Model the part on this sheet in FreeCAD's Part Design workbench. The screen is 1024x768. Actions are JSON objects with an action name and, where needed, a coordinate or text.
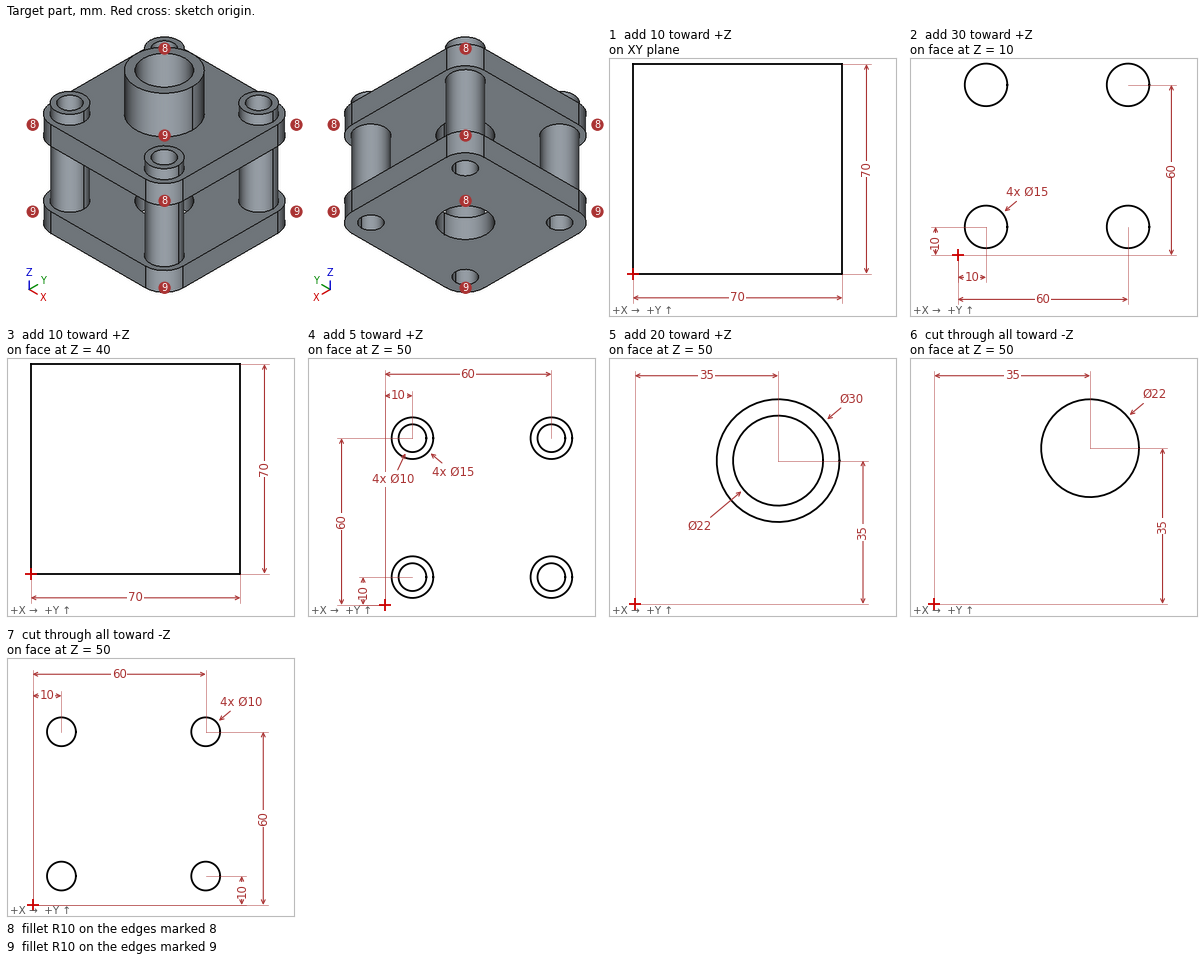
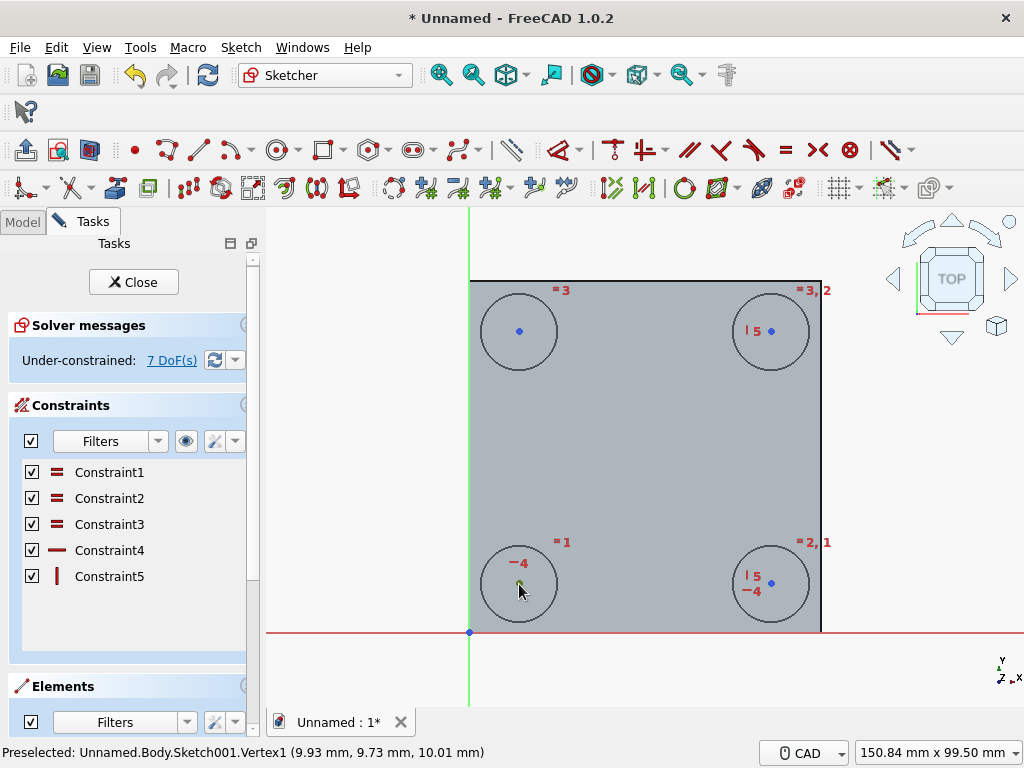
{"action": "left_click", "coordinate": [519, 332]}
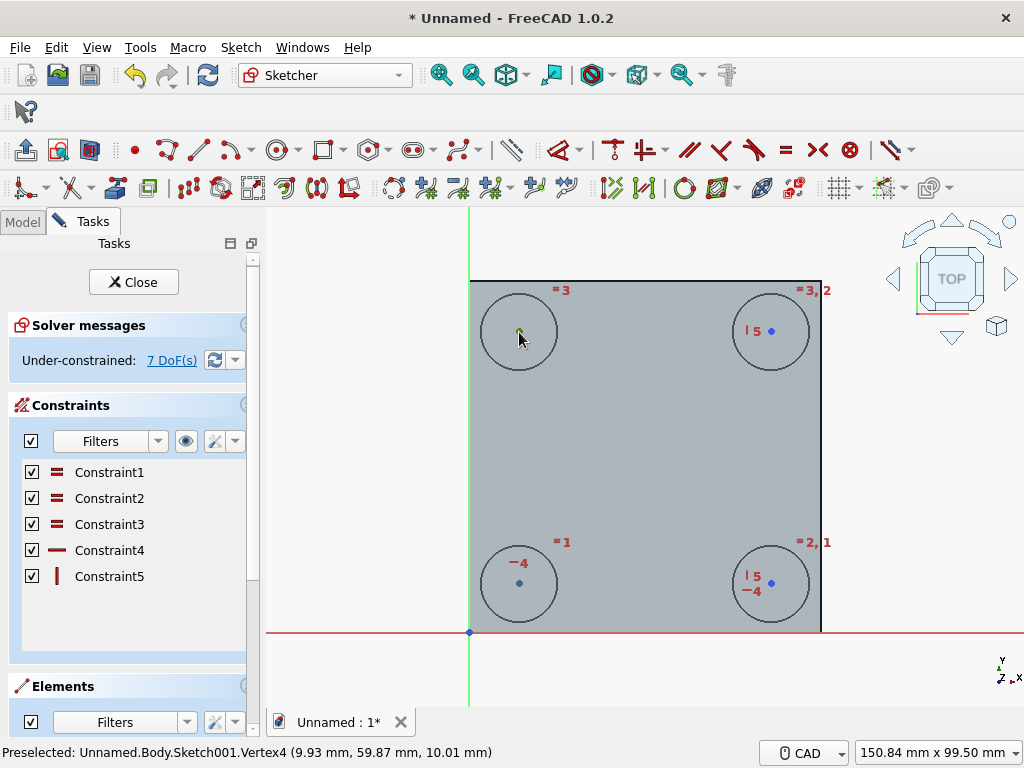
{"action": "key", "text": "v"}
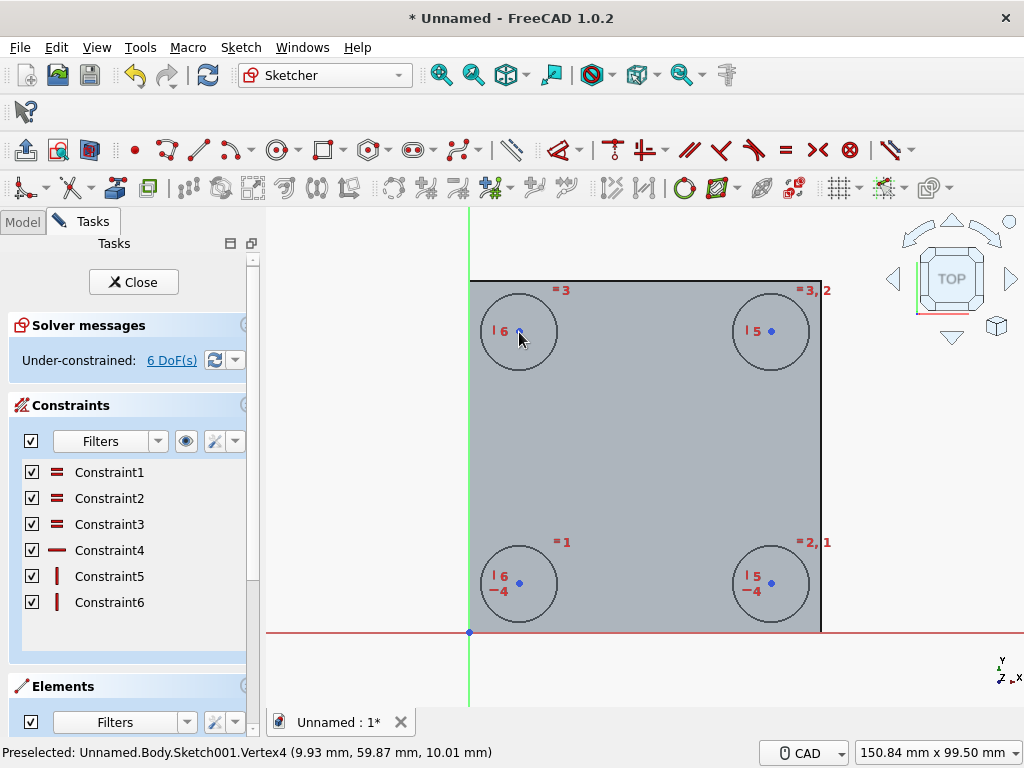
{"action": "left_click", "coordinate": [771, 332]}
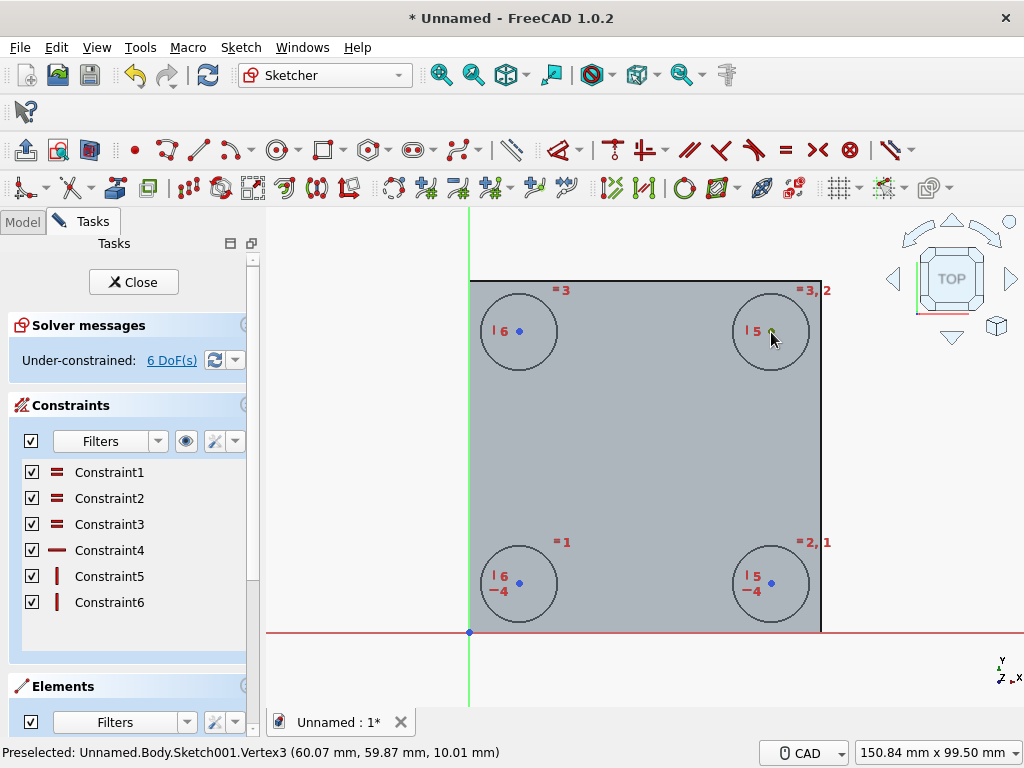
{"action": "left_click", "coordinate": [519, 332]}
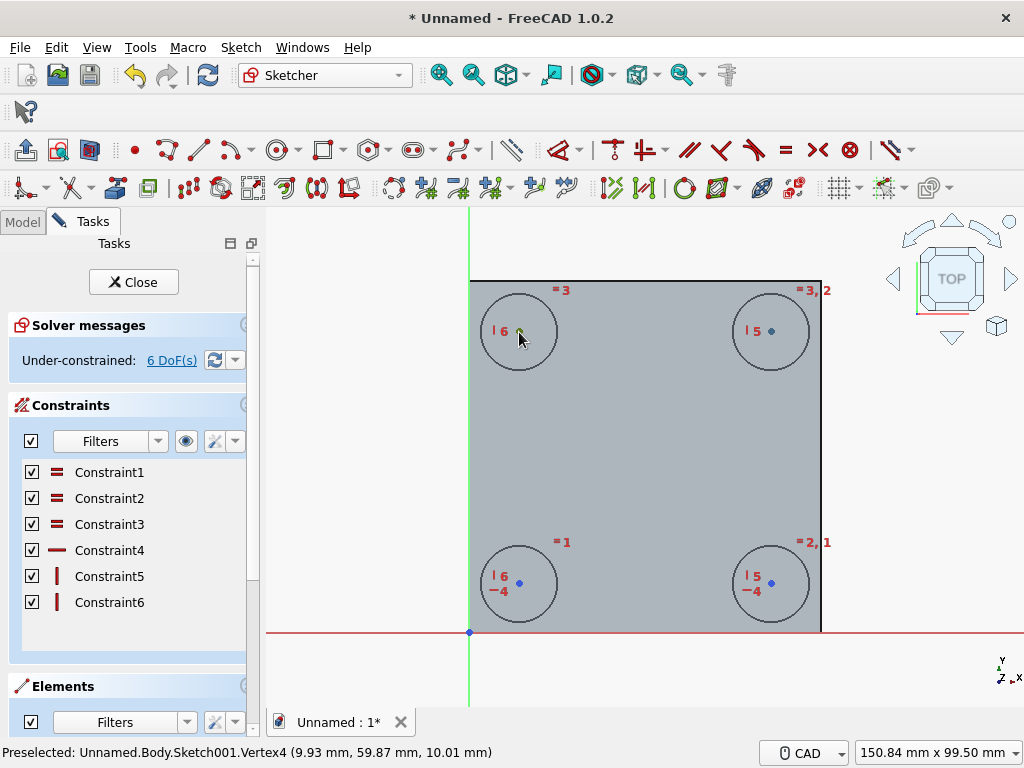
{"action": "key", "text": "h"}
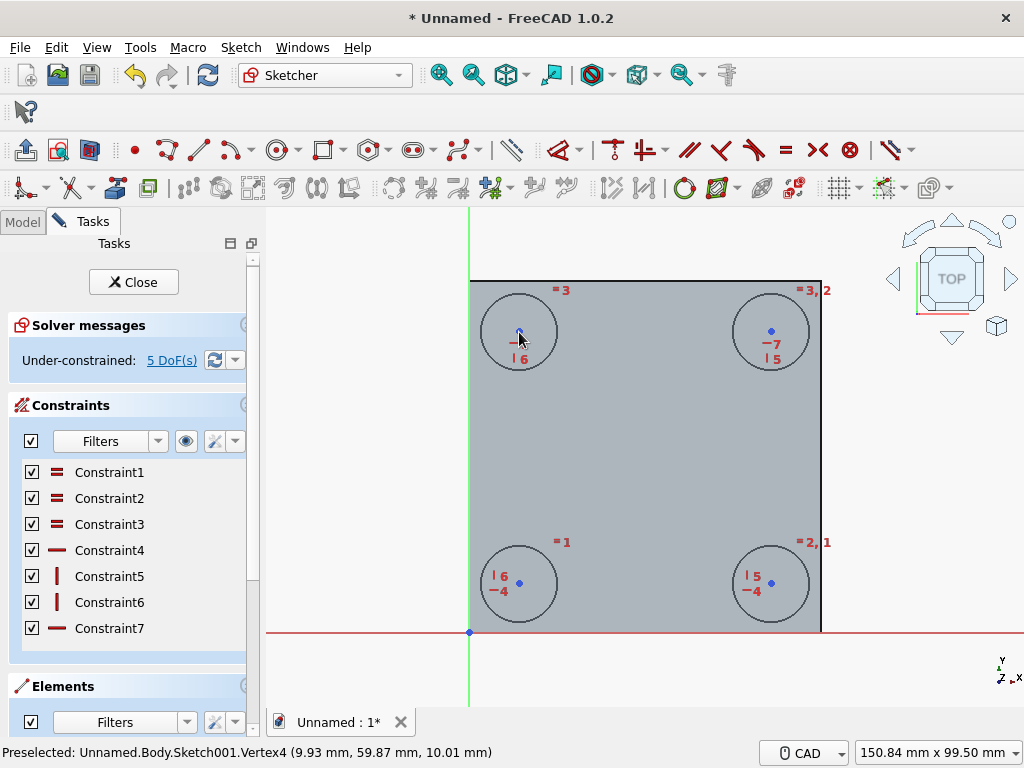
{"action": "key", "text": "d"}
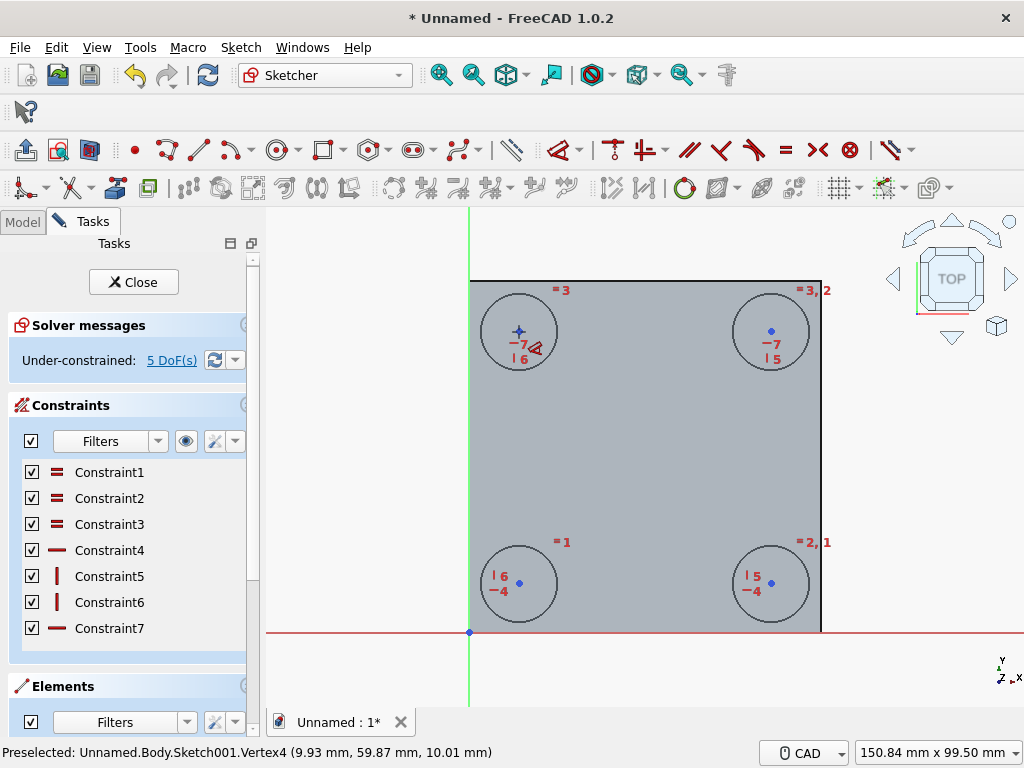
{"action": "left_click", "coordinate": [546, 557]}
{"action": "left_click", "coordinate": [569, 534]}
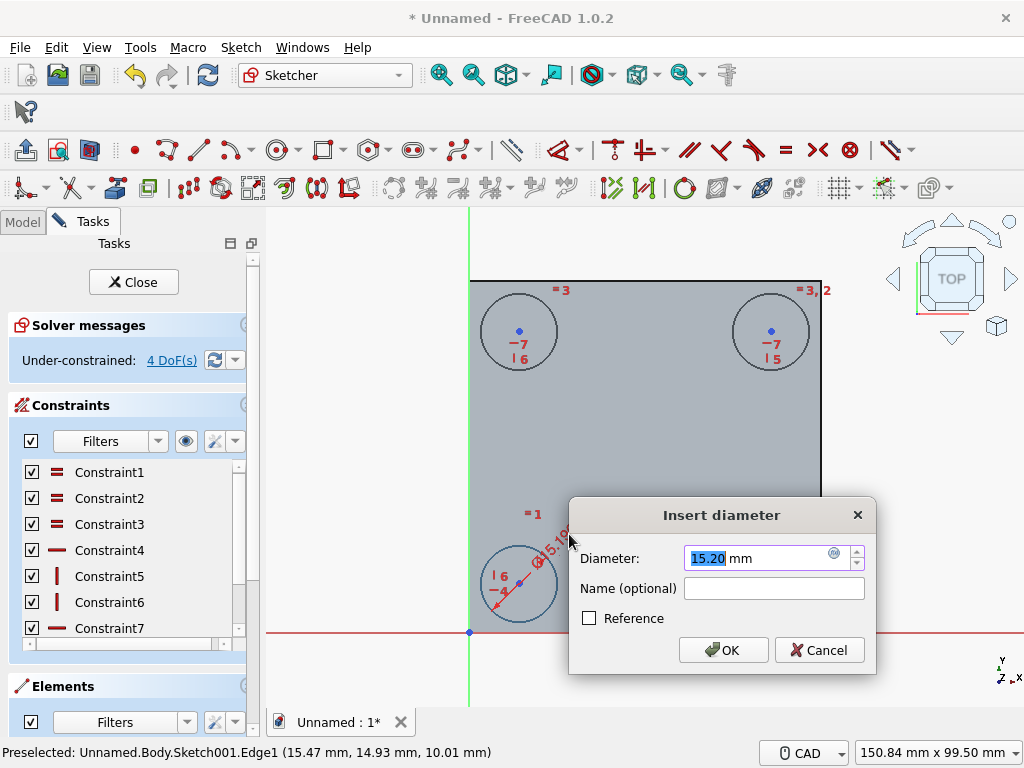
{"action": "type", "text": "15"}
{"action": "key", "text": "Return"}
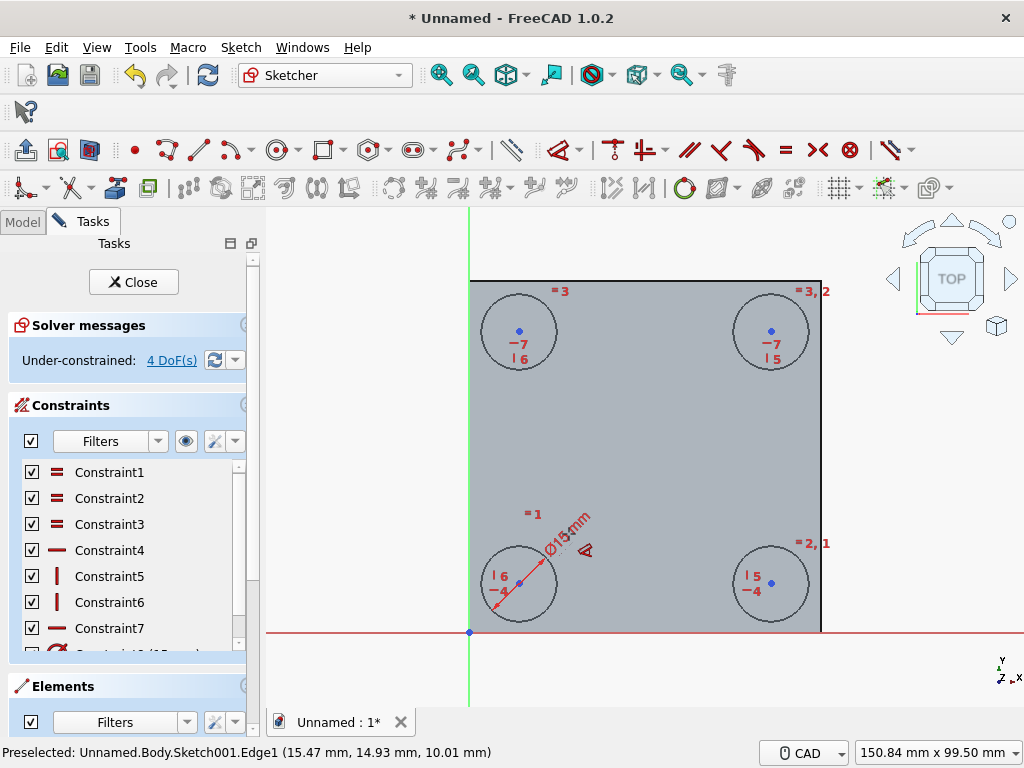
{"action": "left_click", "coordinate": [519, 584]}
{"action": "left_click", "coordinate": [494, 667]}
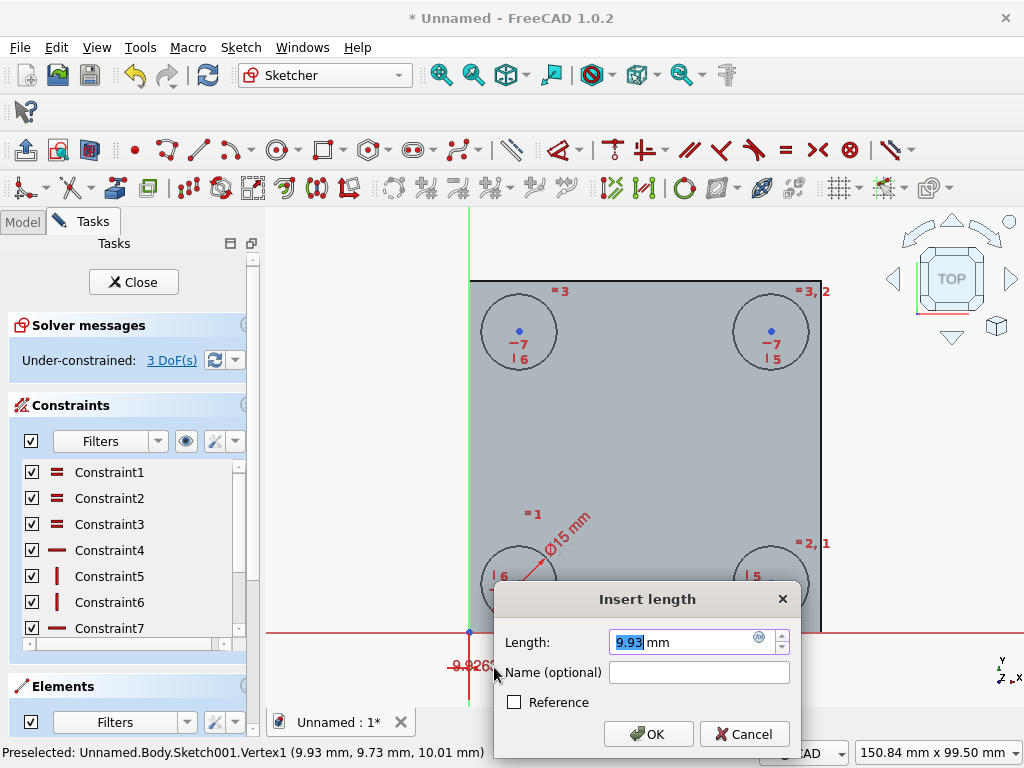
{"action": "type", "text": "10"}
{"action": "key", "text": "Return"}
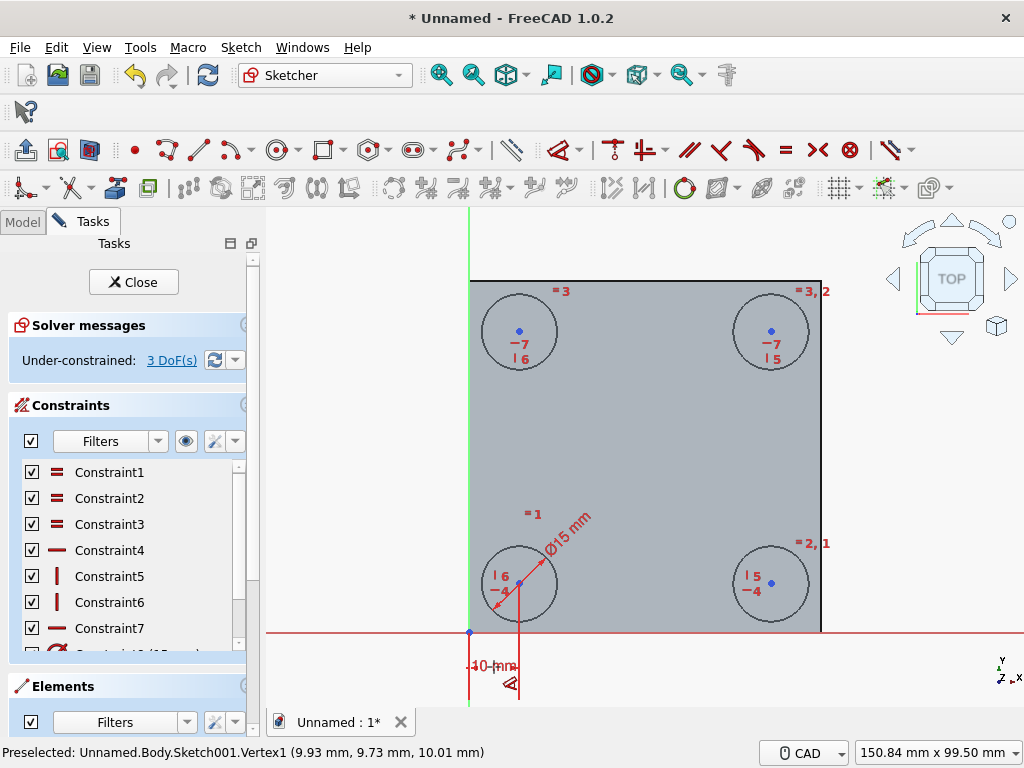
{"action": "left_click", "coordinate": [519, 584]}
{"action": "left_click", "coordinate": [435, 608]}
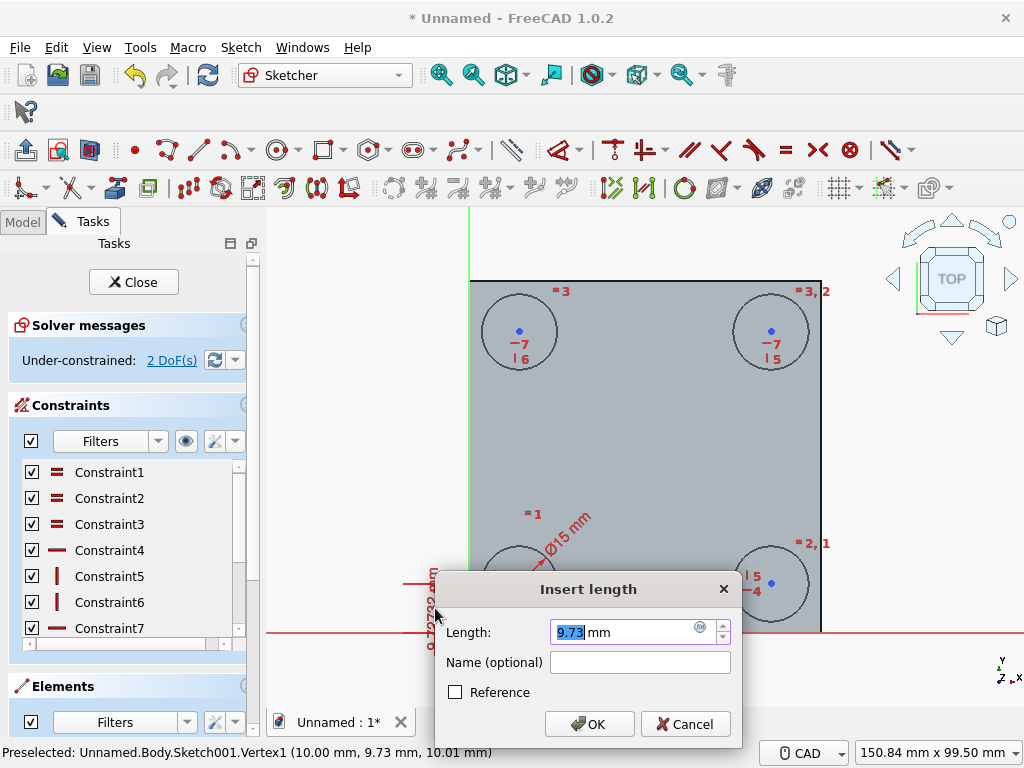
{"action": "type", "text": "10"}
{"action": "key", "text": "Return"}